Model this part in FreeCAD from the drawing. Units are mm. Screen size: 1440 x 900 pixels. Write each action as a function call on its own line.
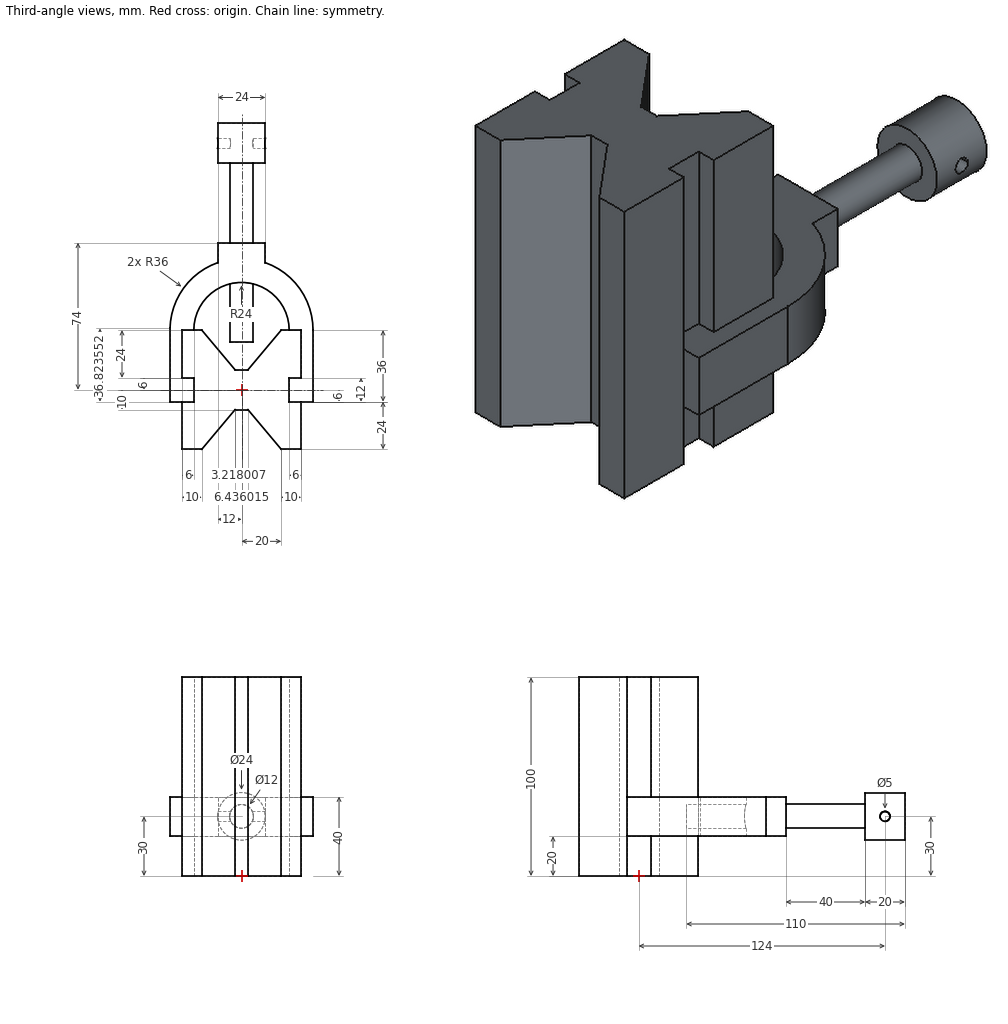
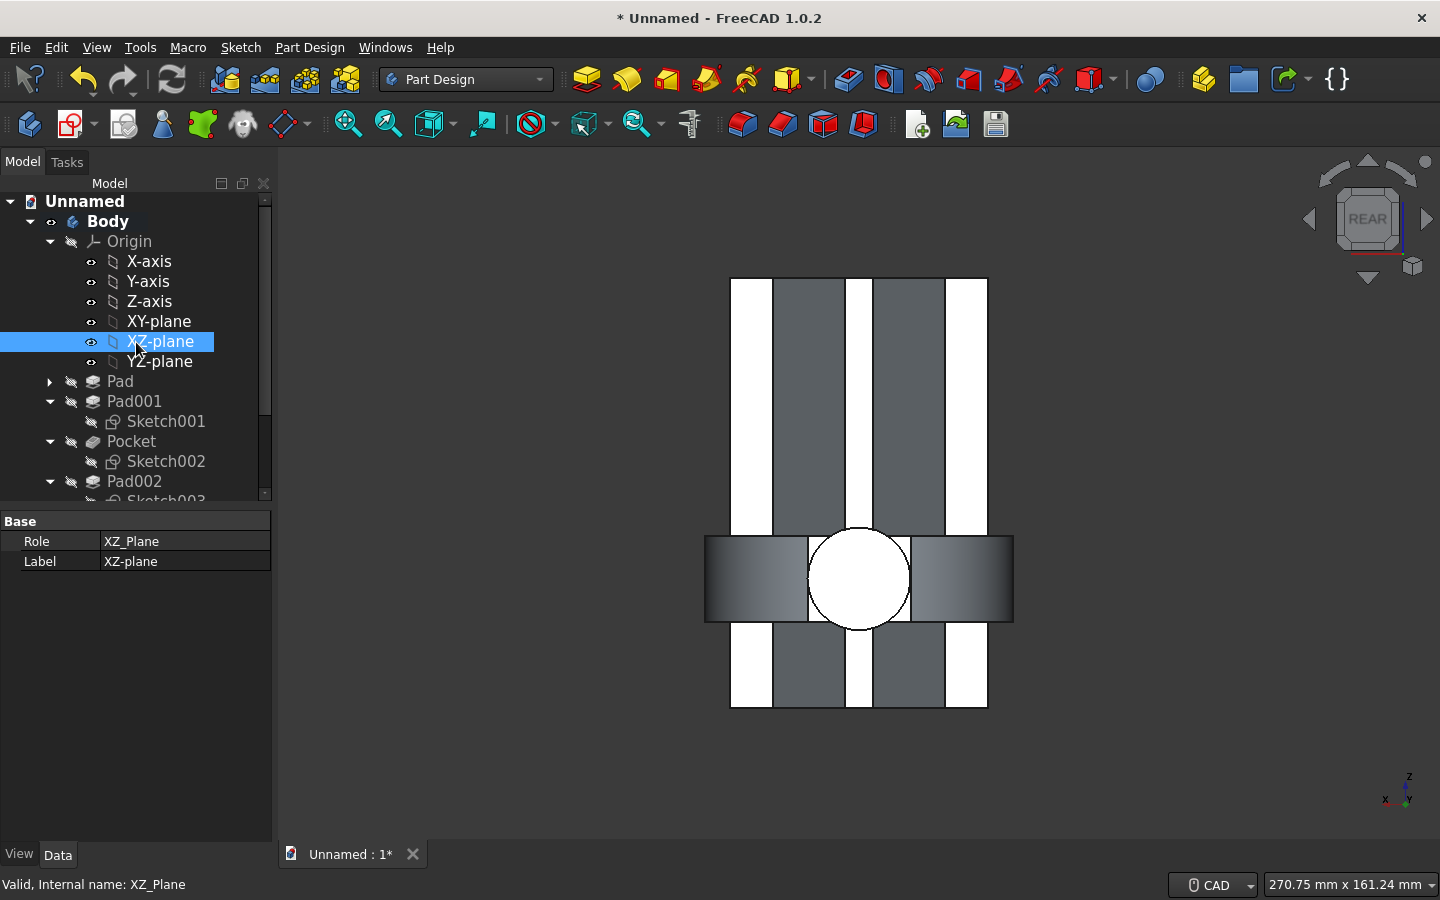
click(284, 124)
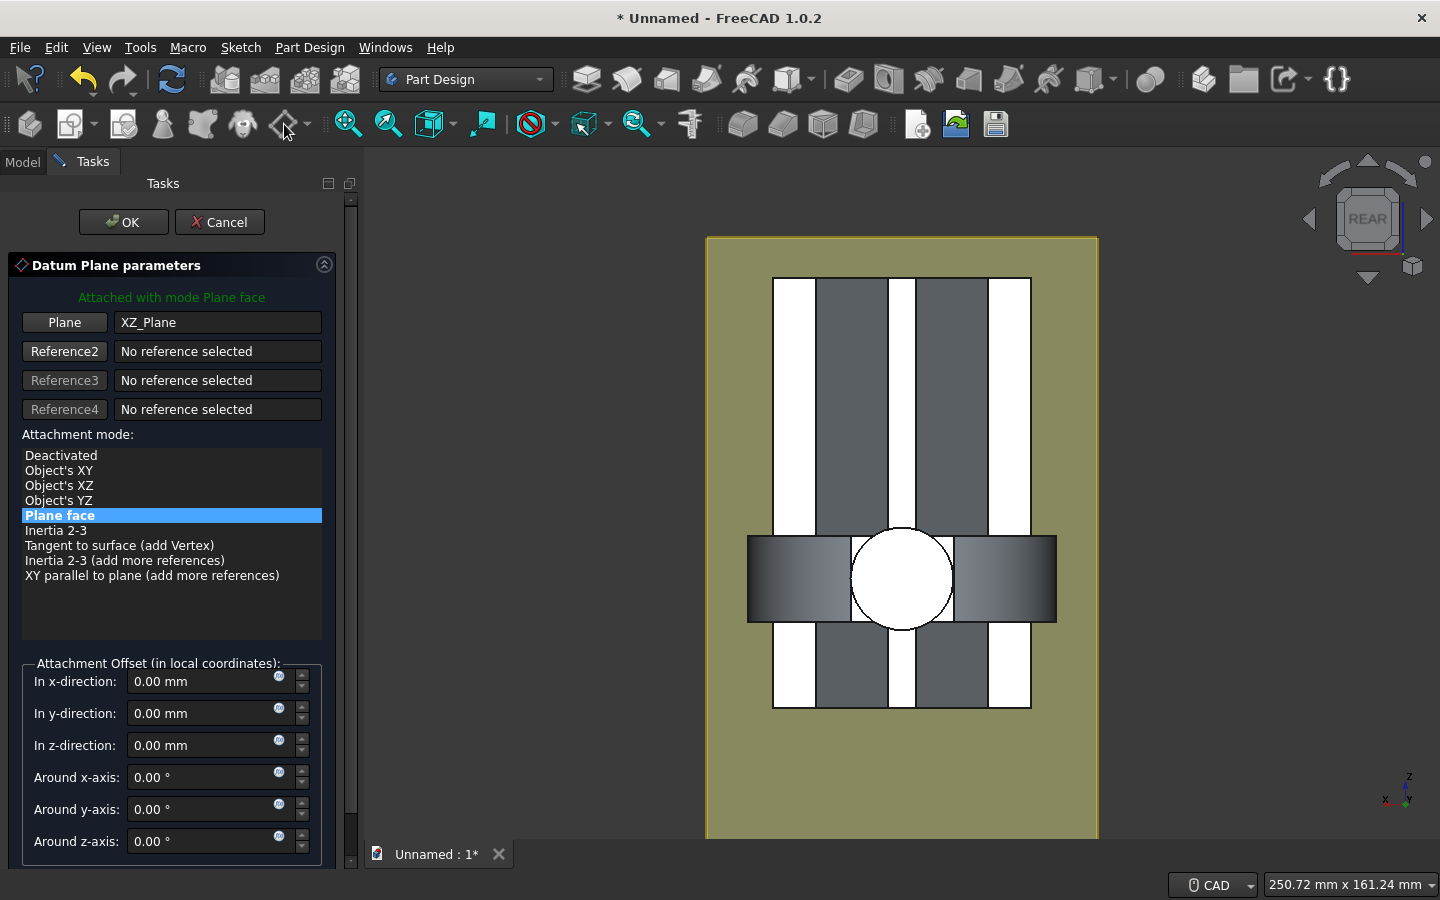
triple_click(210, 745)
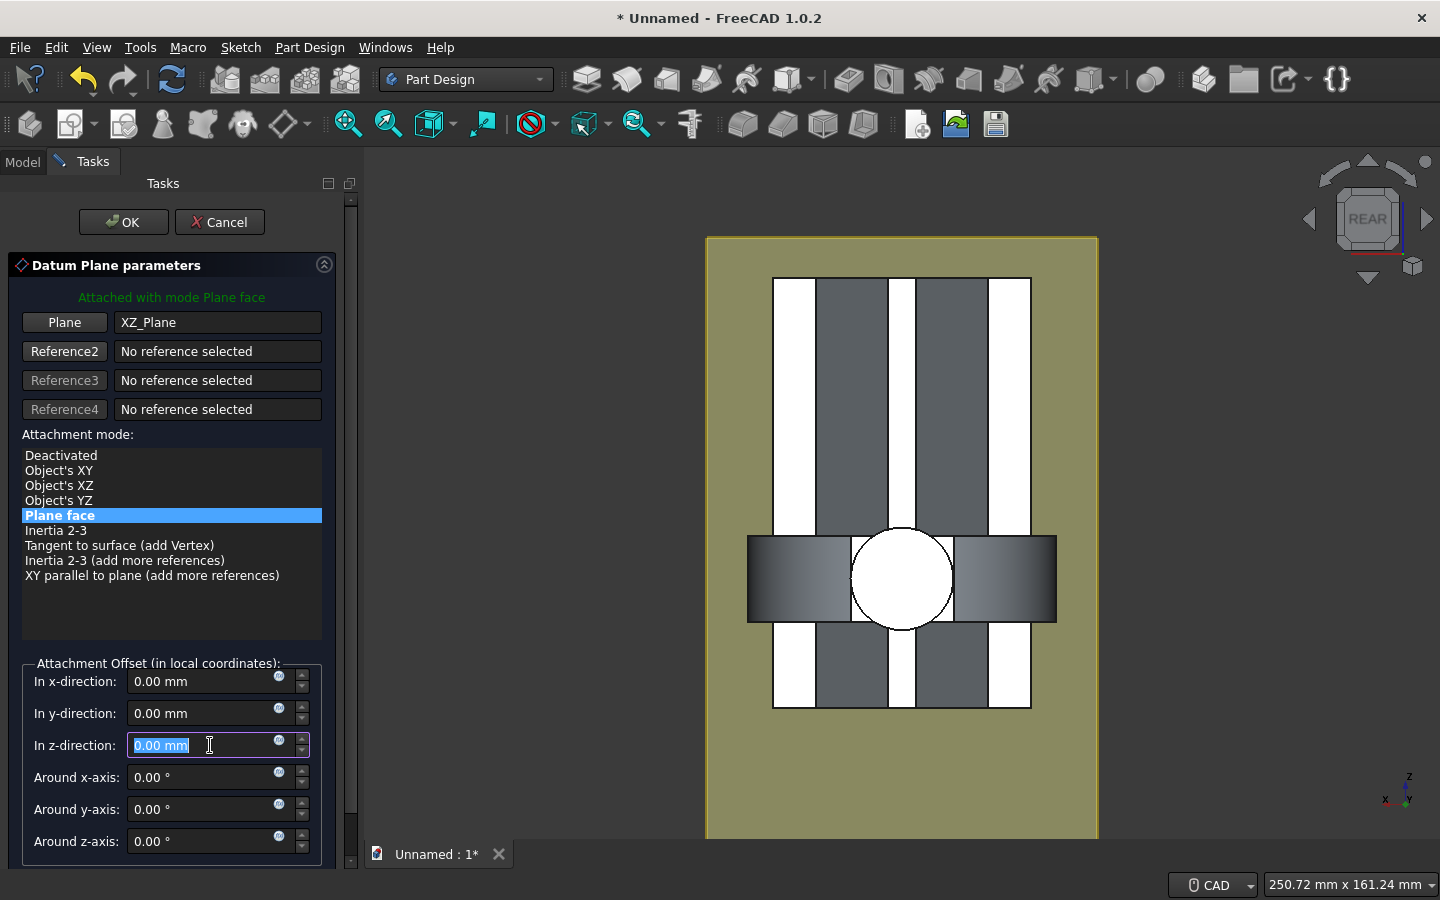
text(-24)
key(Tab)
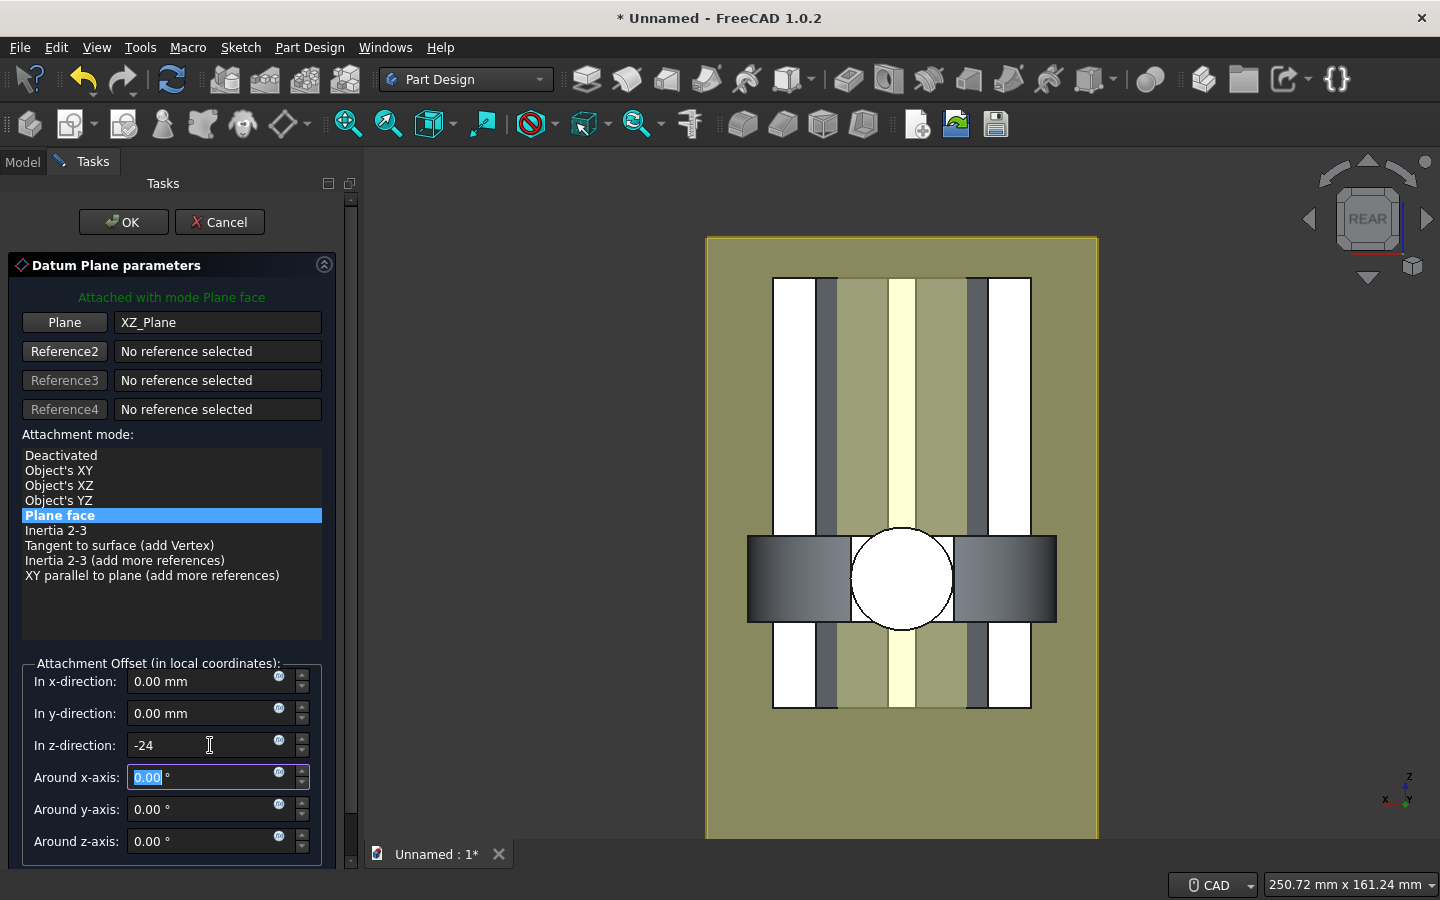
click(124, 222)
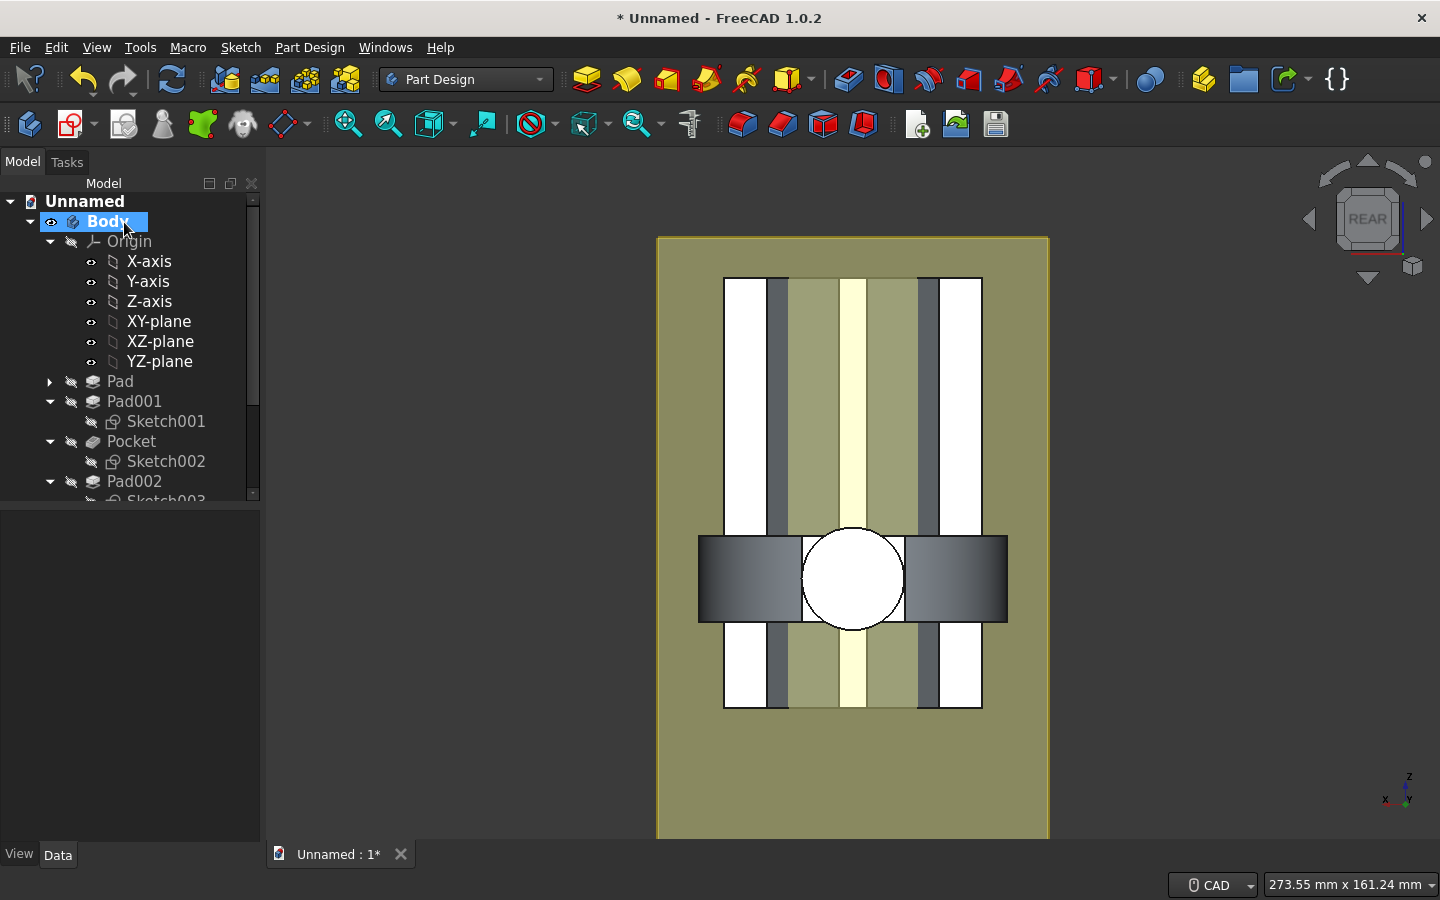
scroll(100, 337, down, 3)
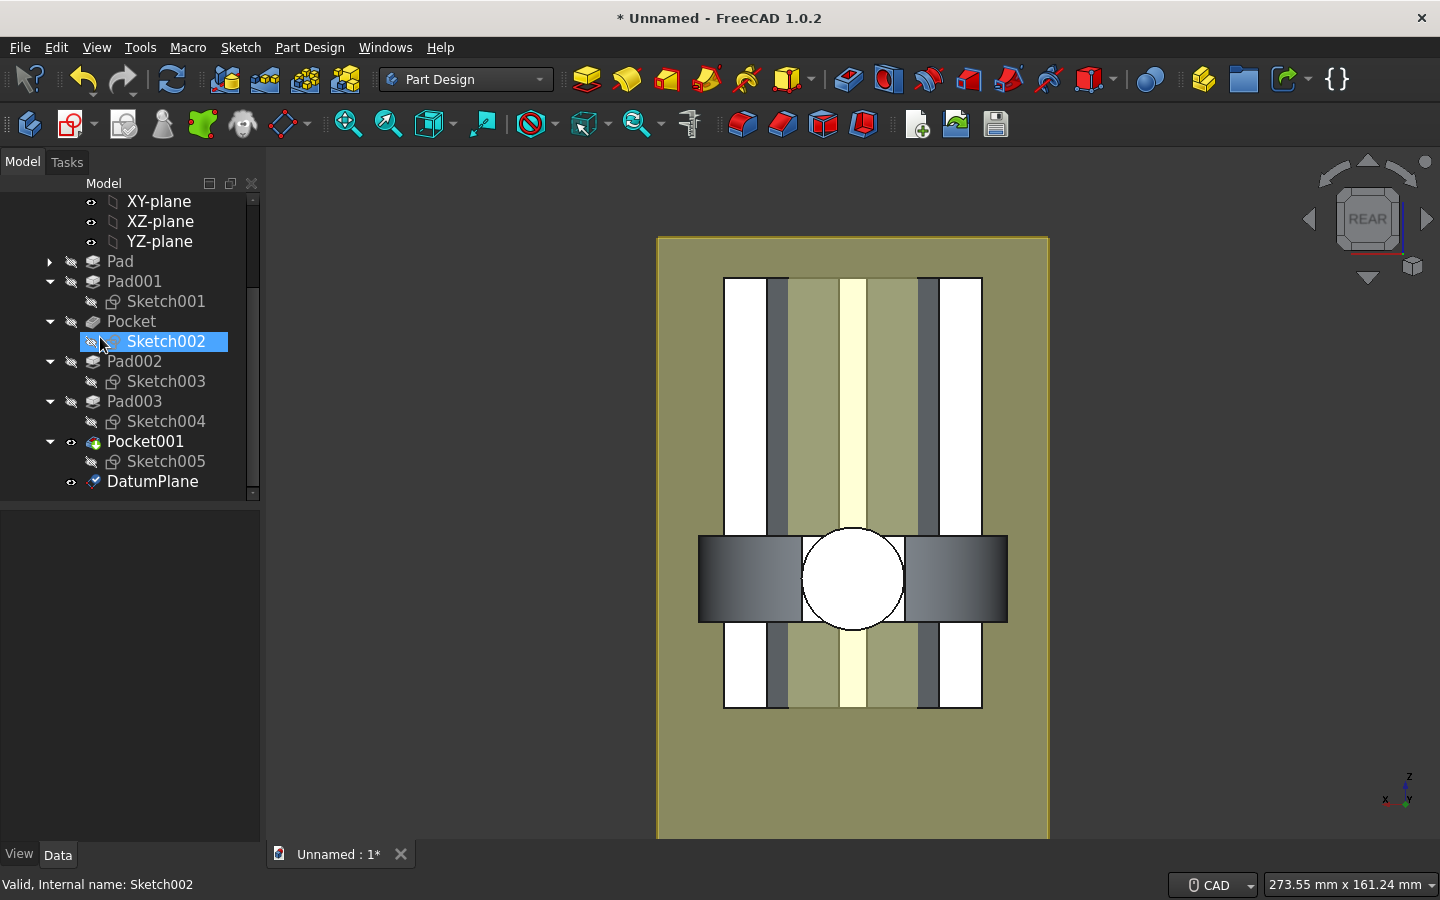
click(116, 482)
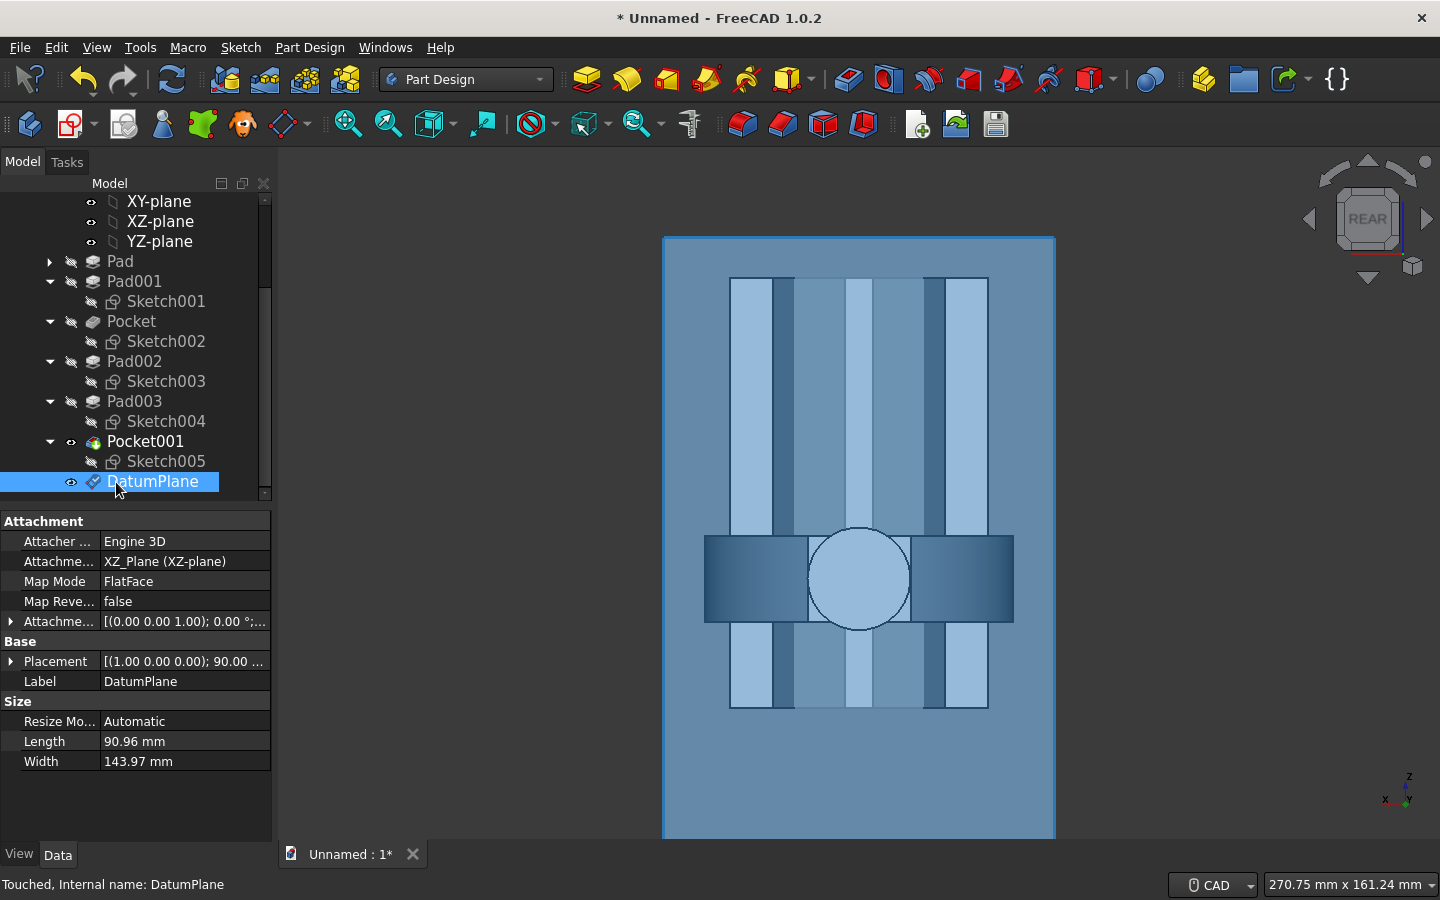
click(70, 124)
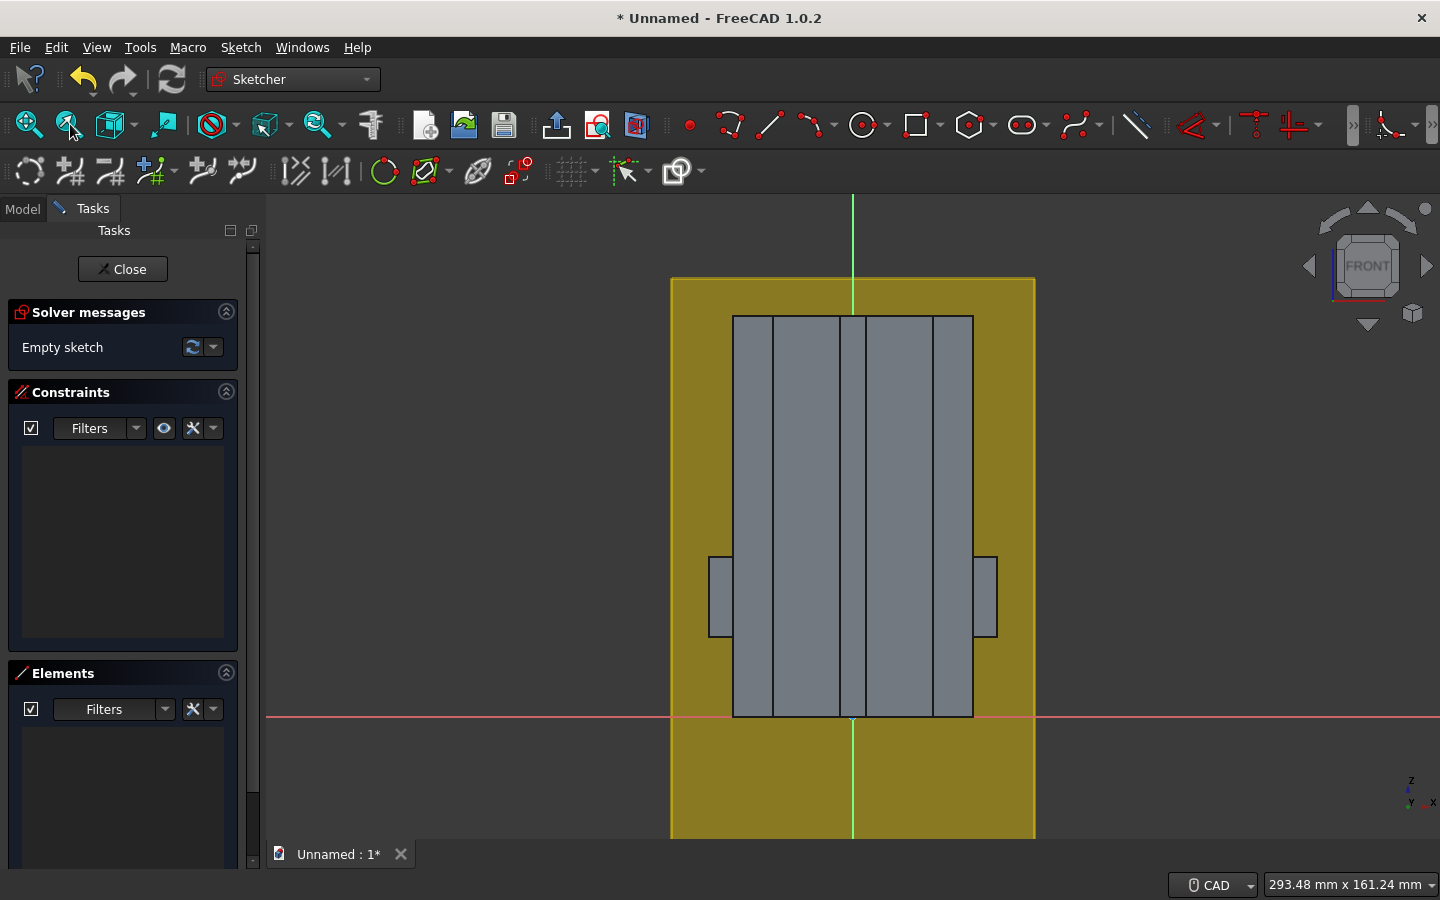
click(638, 126)